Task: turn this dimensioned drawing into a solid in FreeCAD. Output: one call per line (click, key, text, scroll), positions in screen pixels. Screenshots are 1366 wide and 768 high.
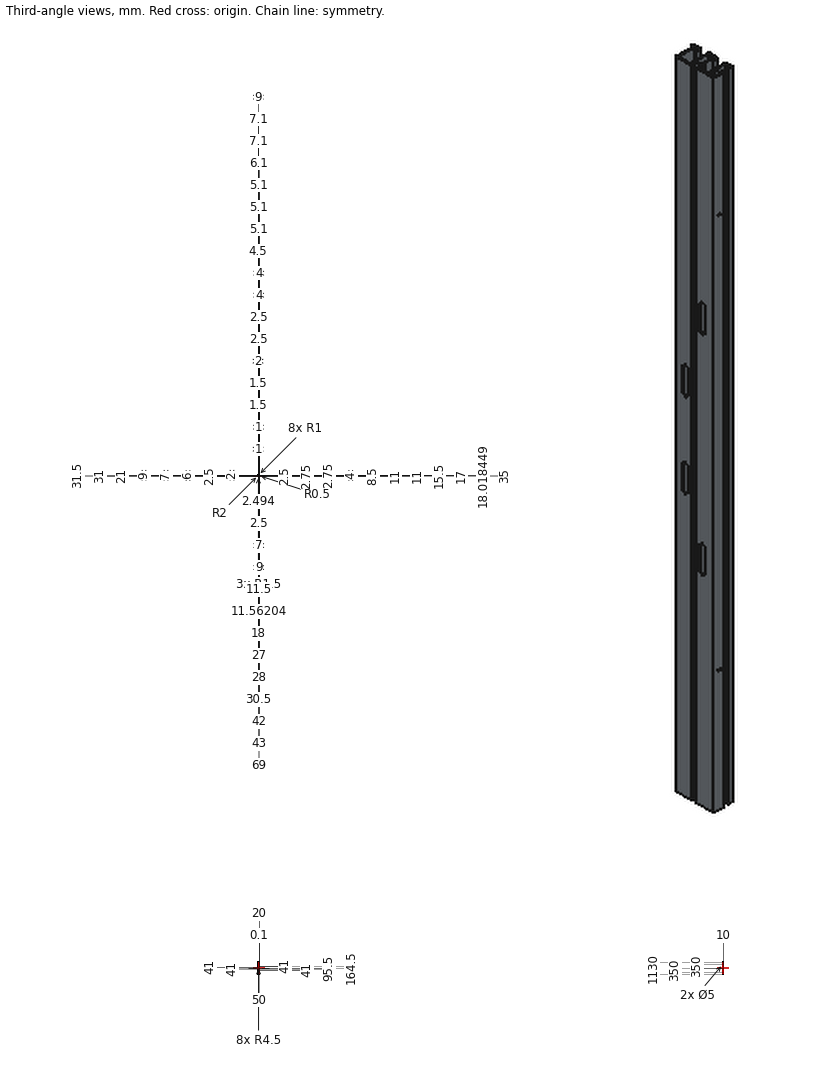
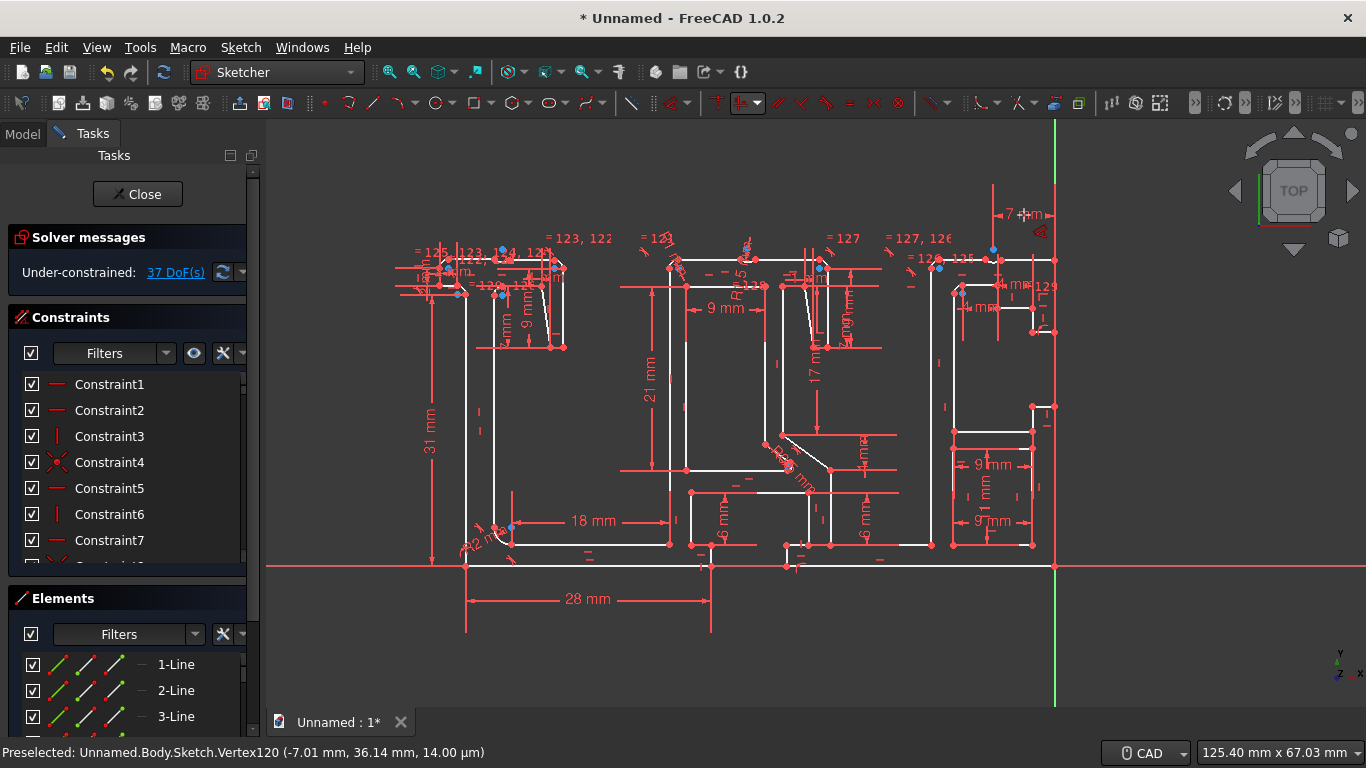
click(800, 260)
click(787, 226)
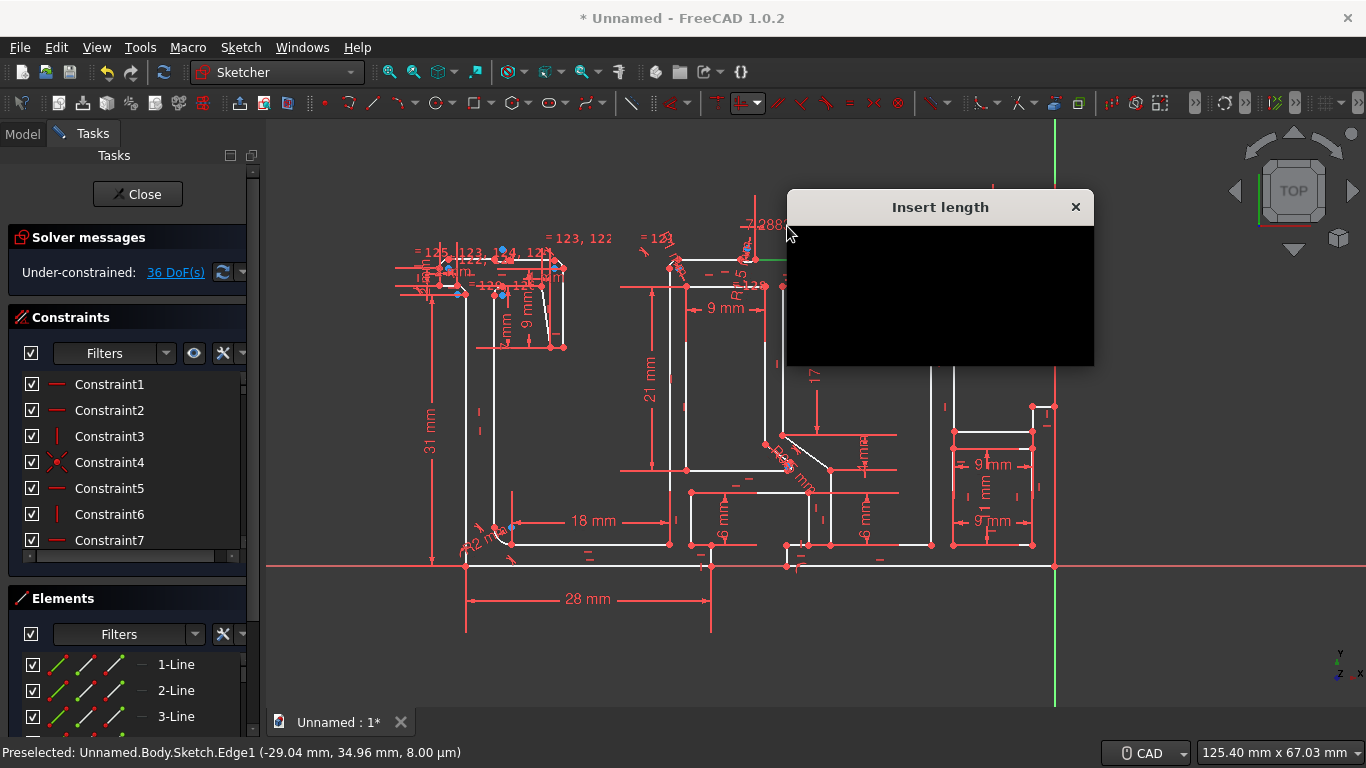
text(7.1)
key(Return)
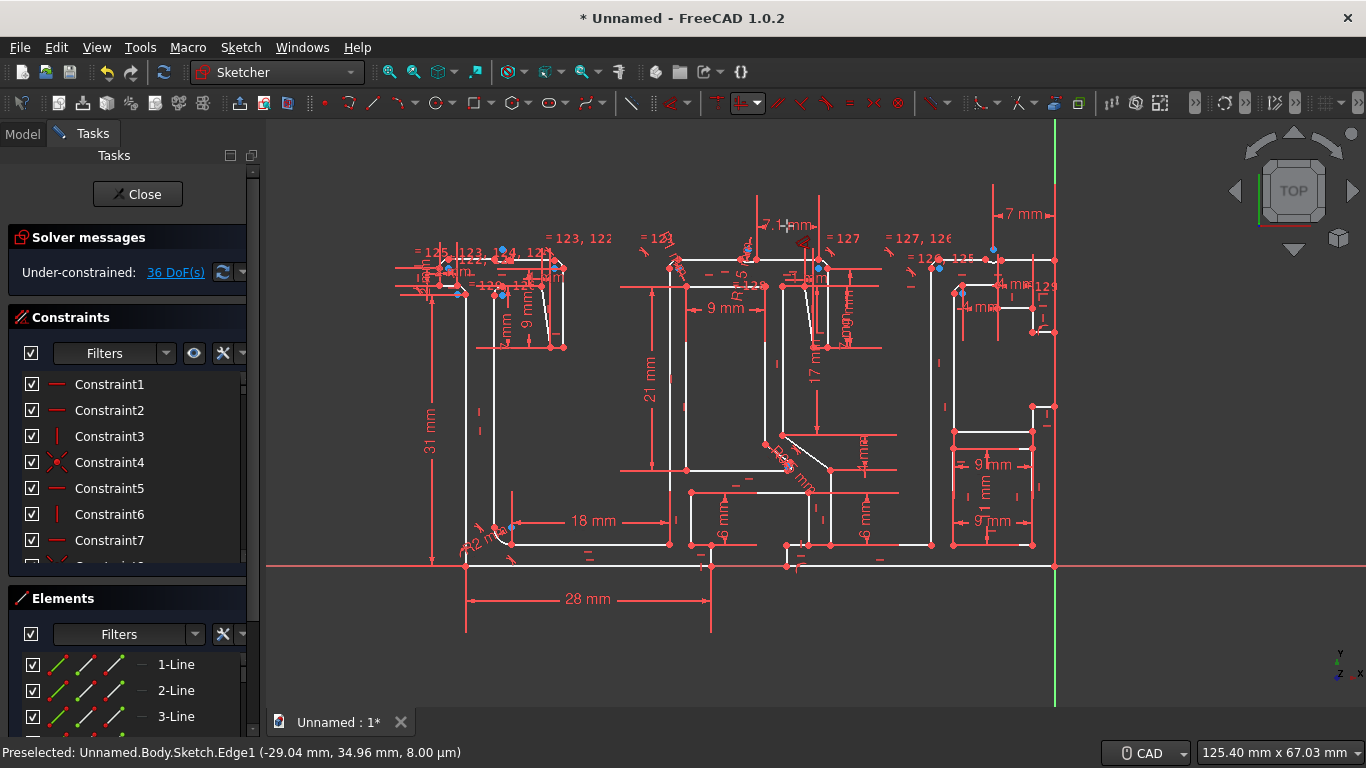
click(722, 259)
click(709, 225)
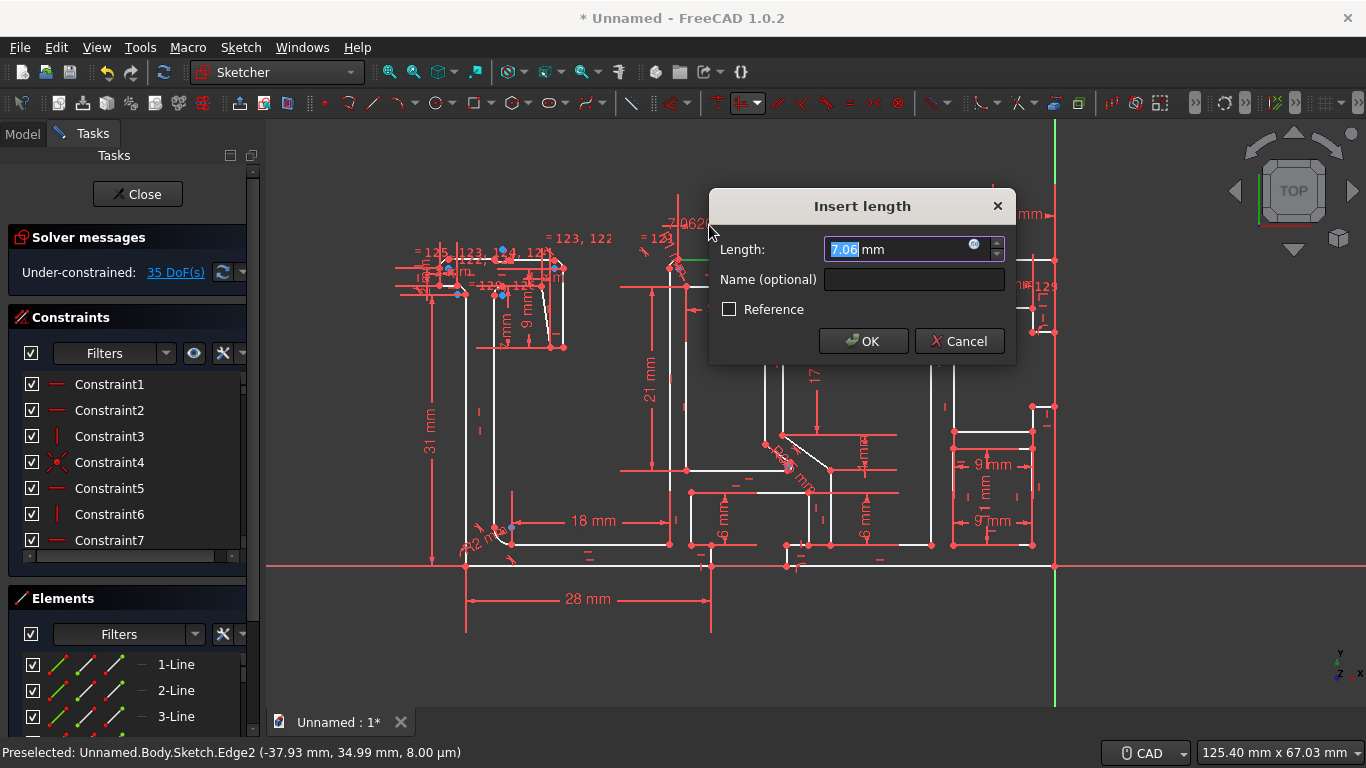
text(7.1)
key(Return)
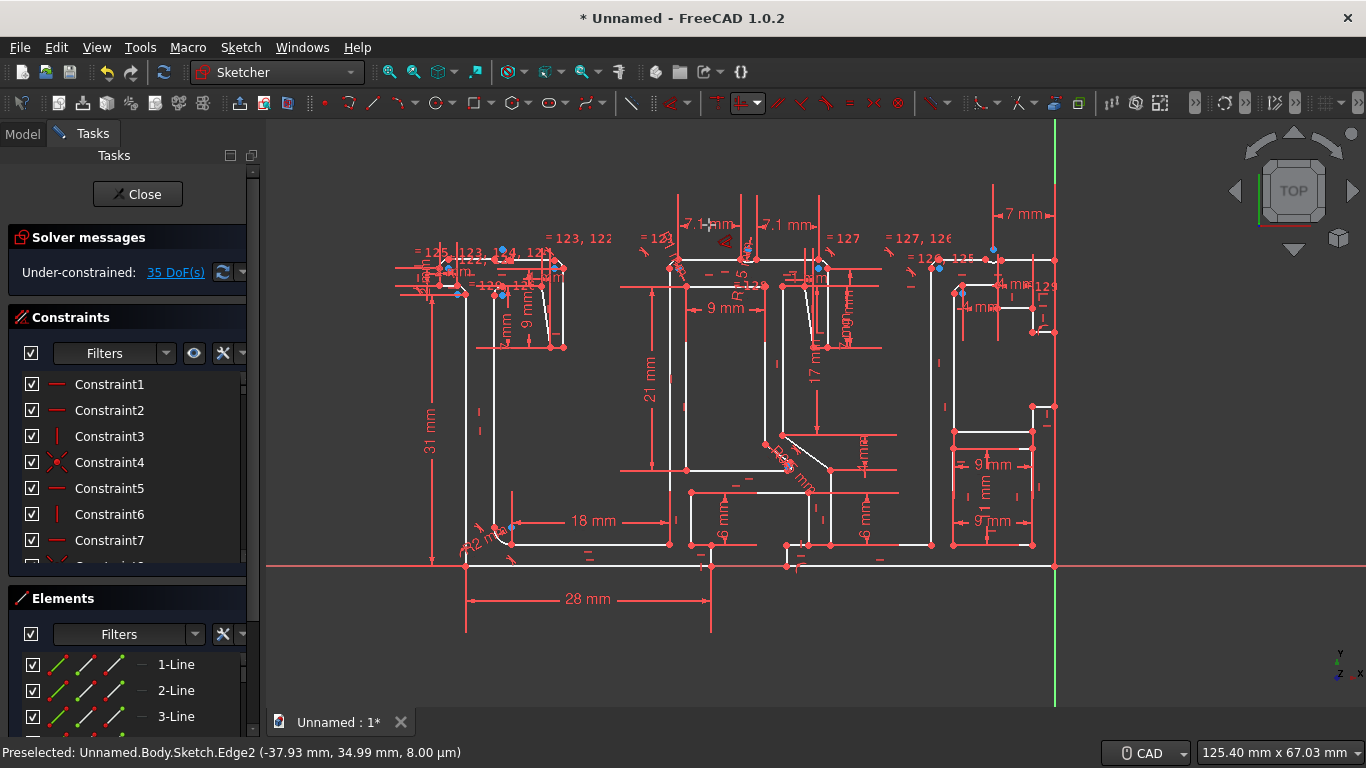
click(515, 286)
click(522, 228)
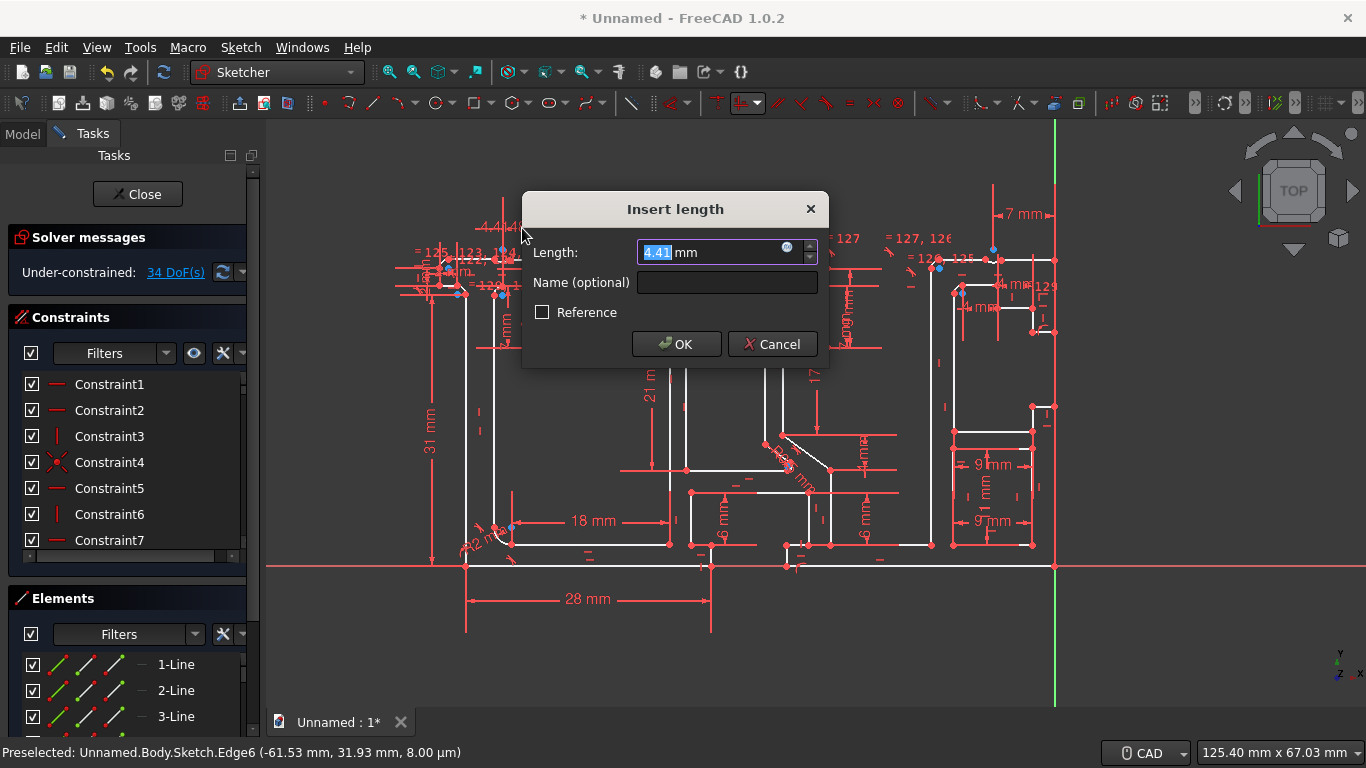
text(4.5)
key(Return)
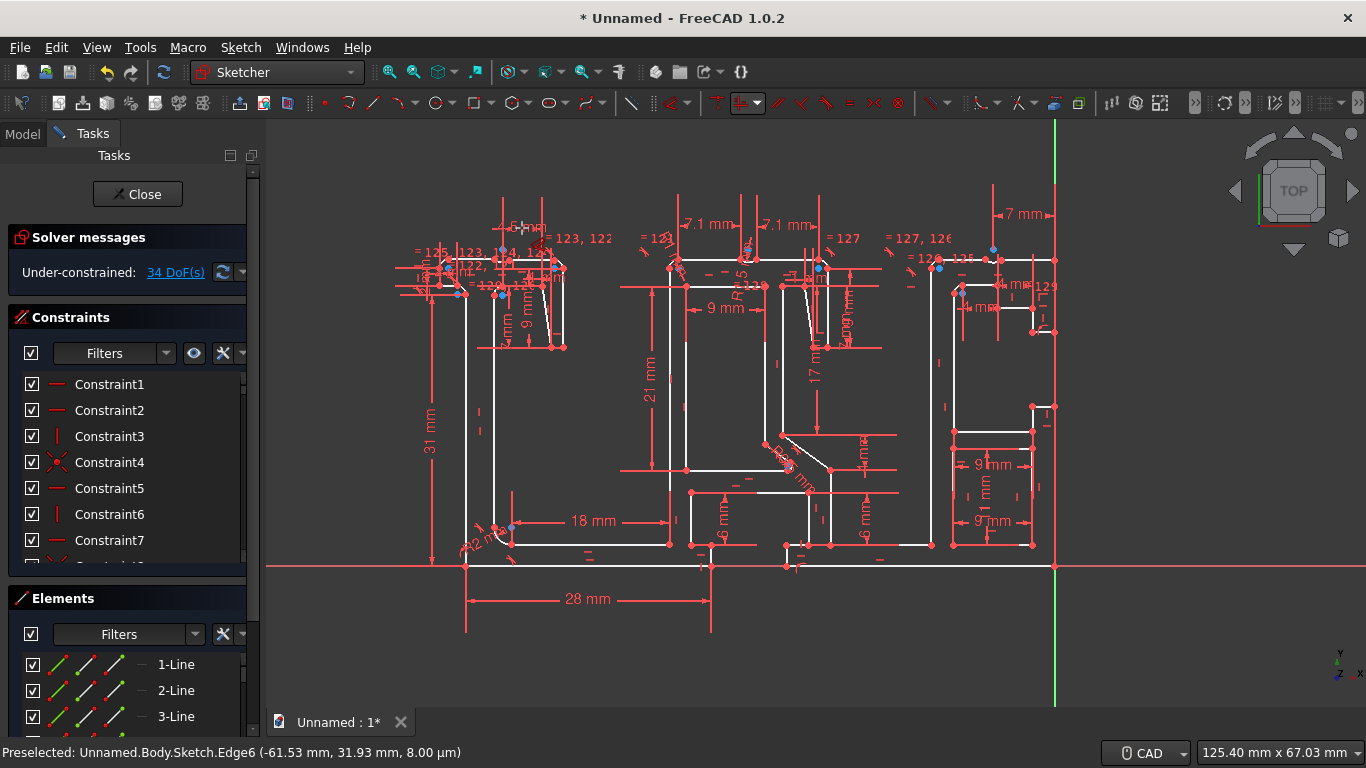
scroll(557, 348, up, 6)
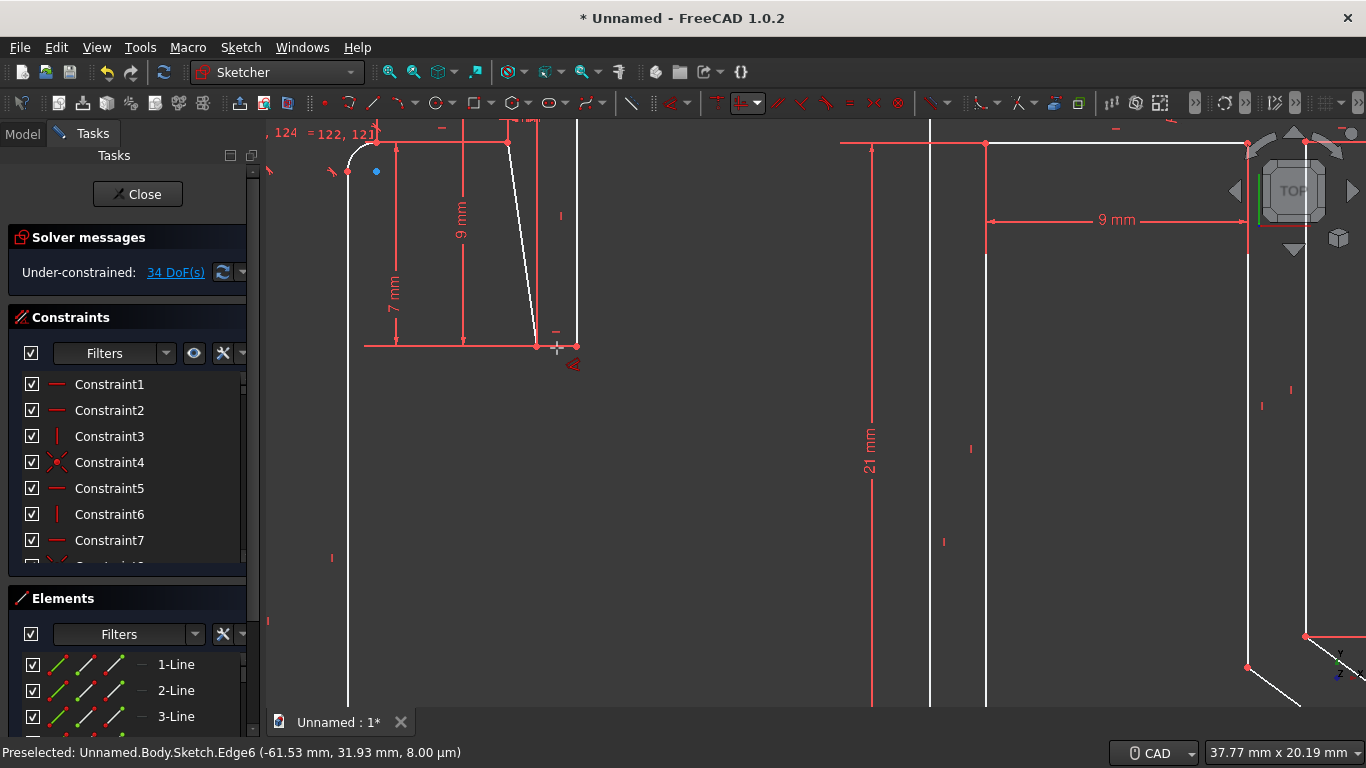
click(557, 346)
click(557, 312)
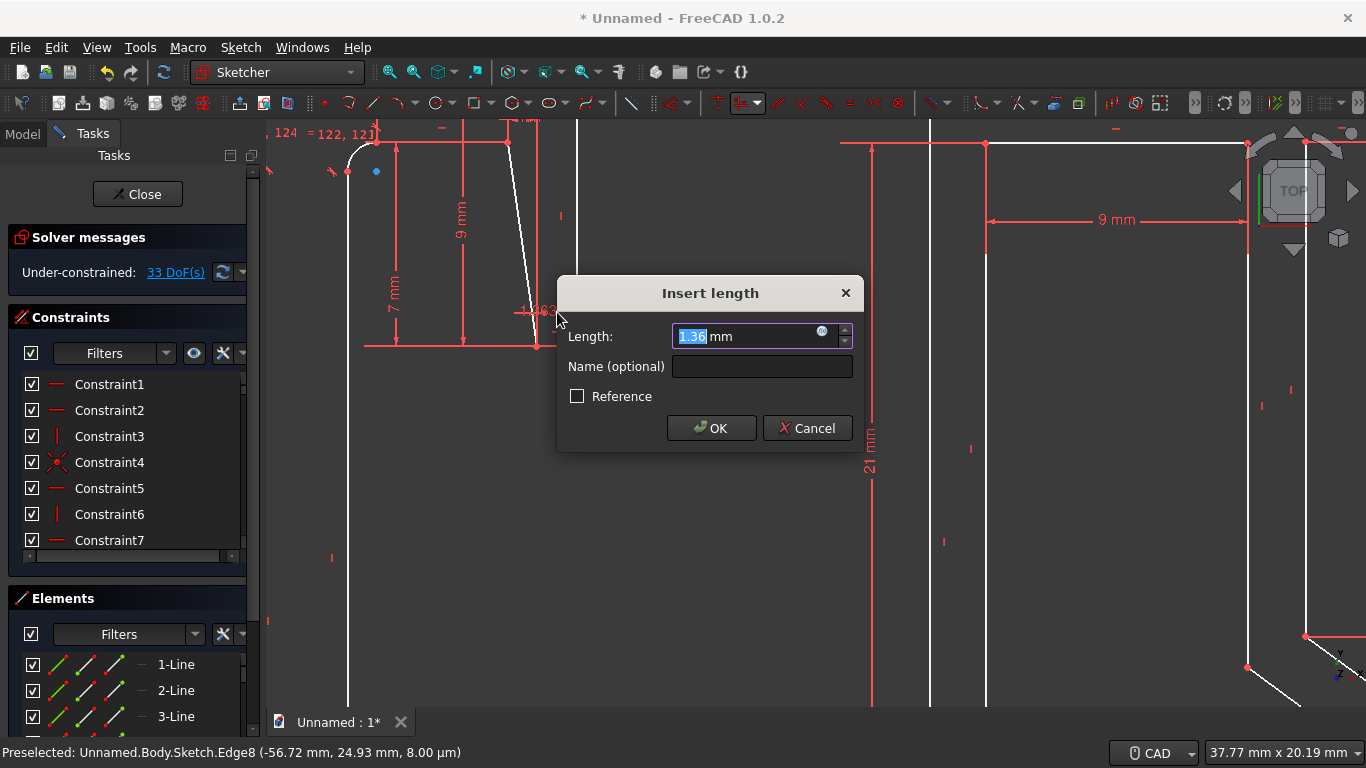
text(1.5)
key(Return)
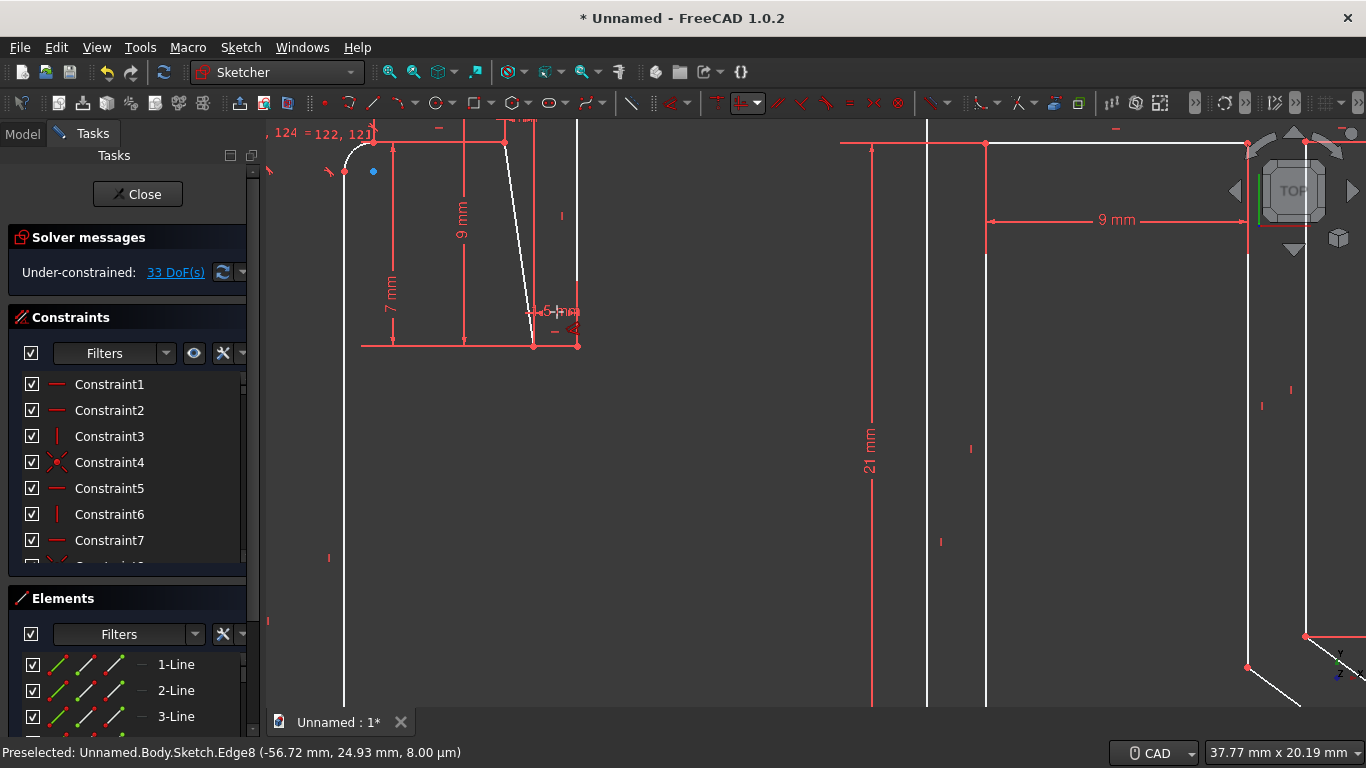
scroll(557, 348, down, 6)